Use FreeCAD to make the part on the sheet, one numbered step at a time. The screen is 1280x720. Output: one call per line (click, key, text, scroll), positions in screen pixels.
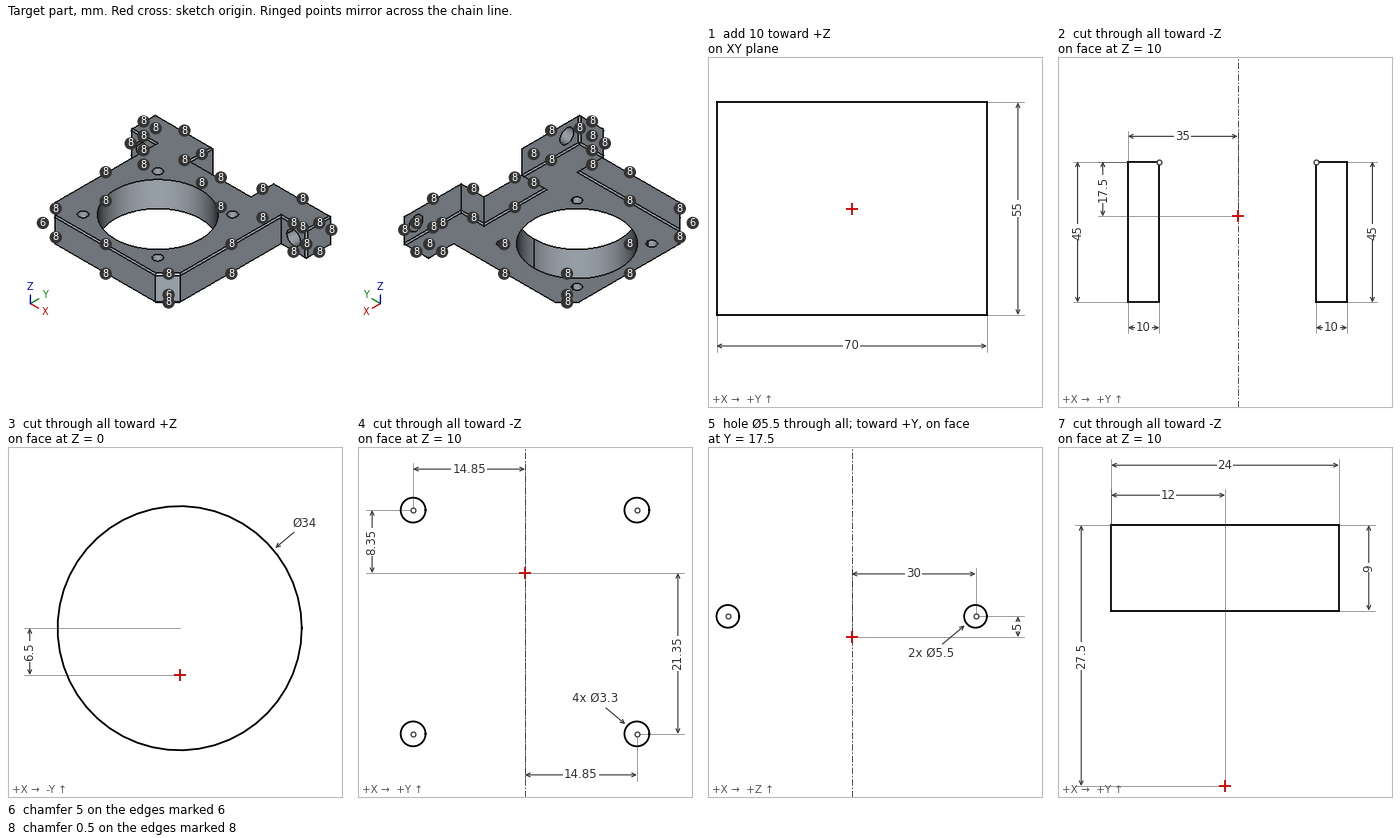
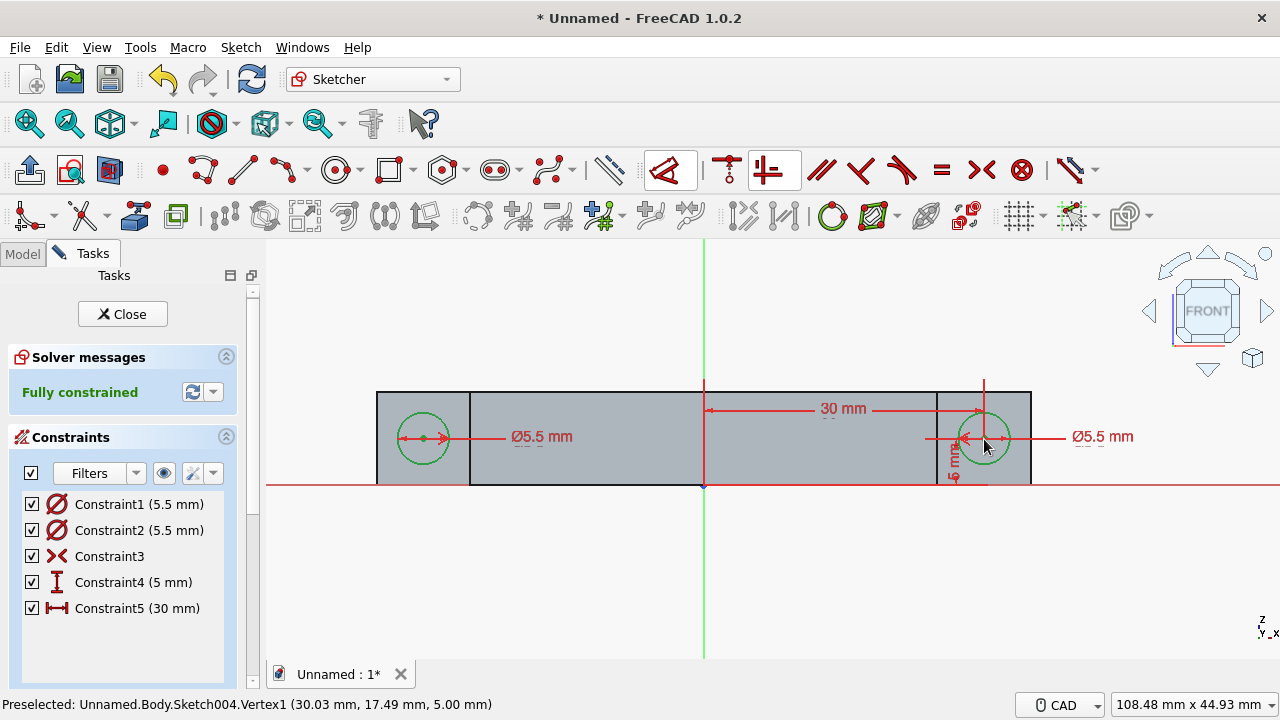
click(123, 314)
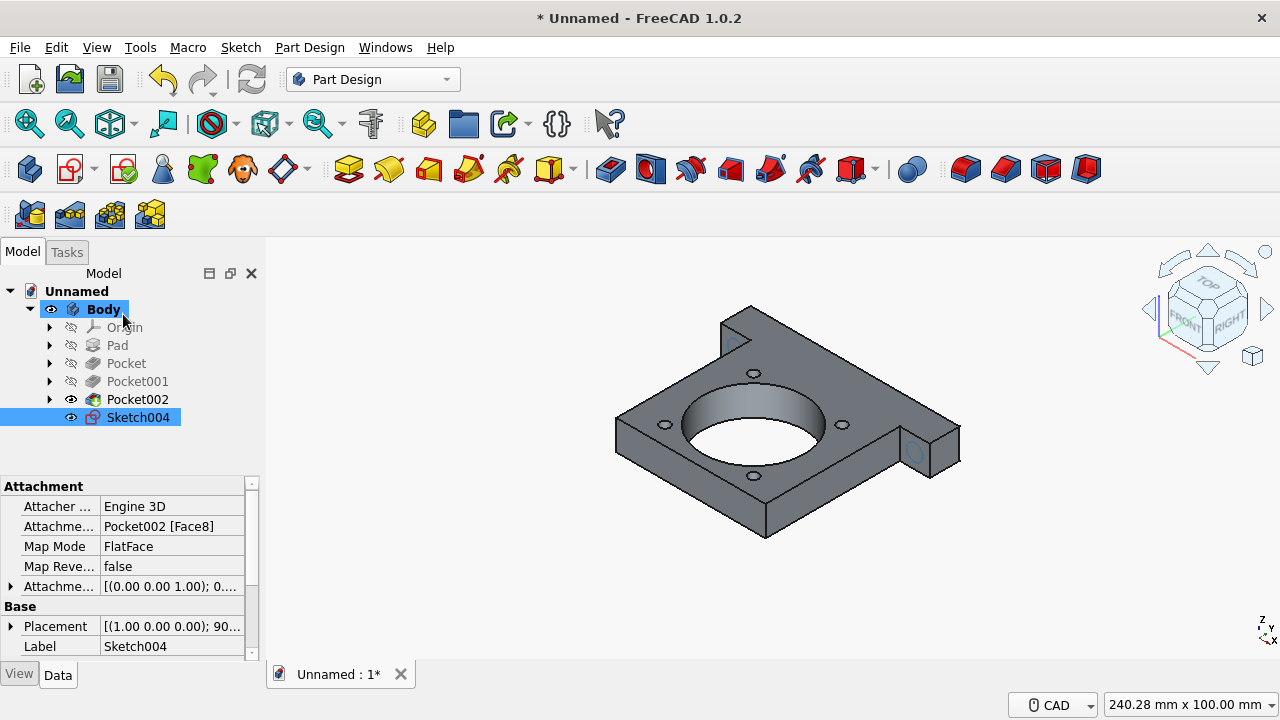
click(652, 170)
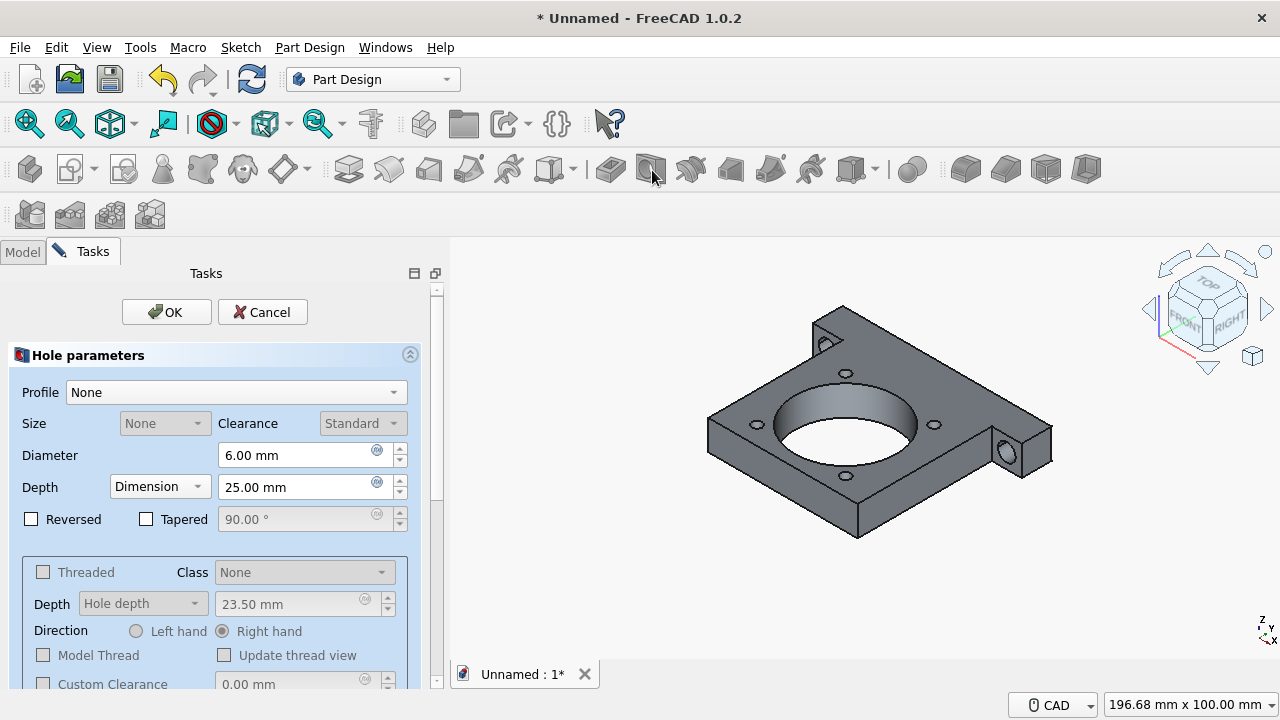
triple_click(305, 455)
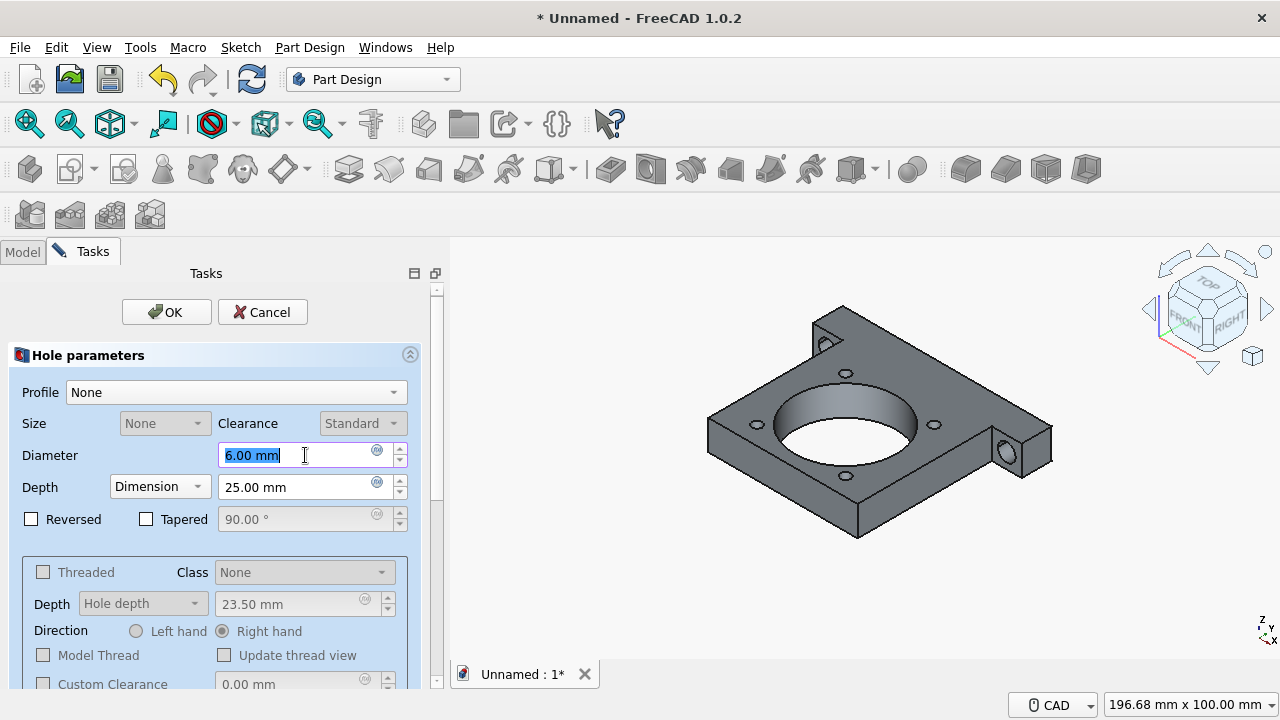
text(5.5)
key(Tab)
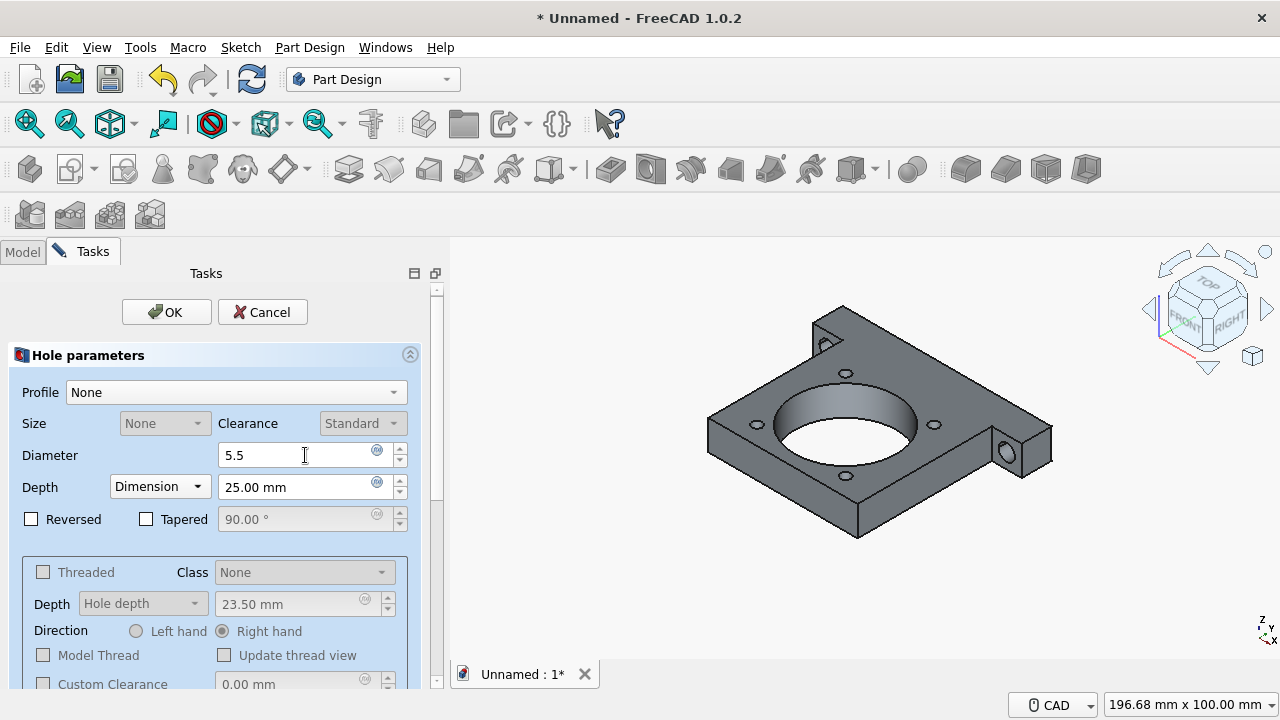
click(161, 486)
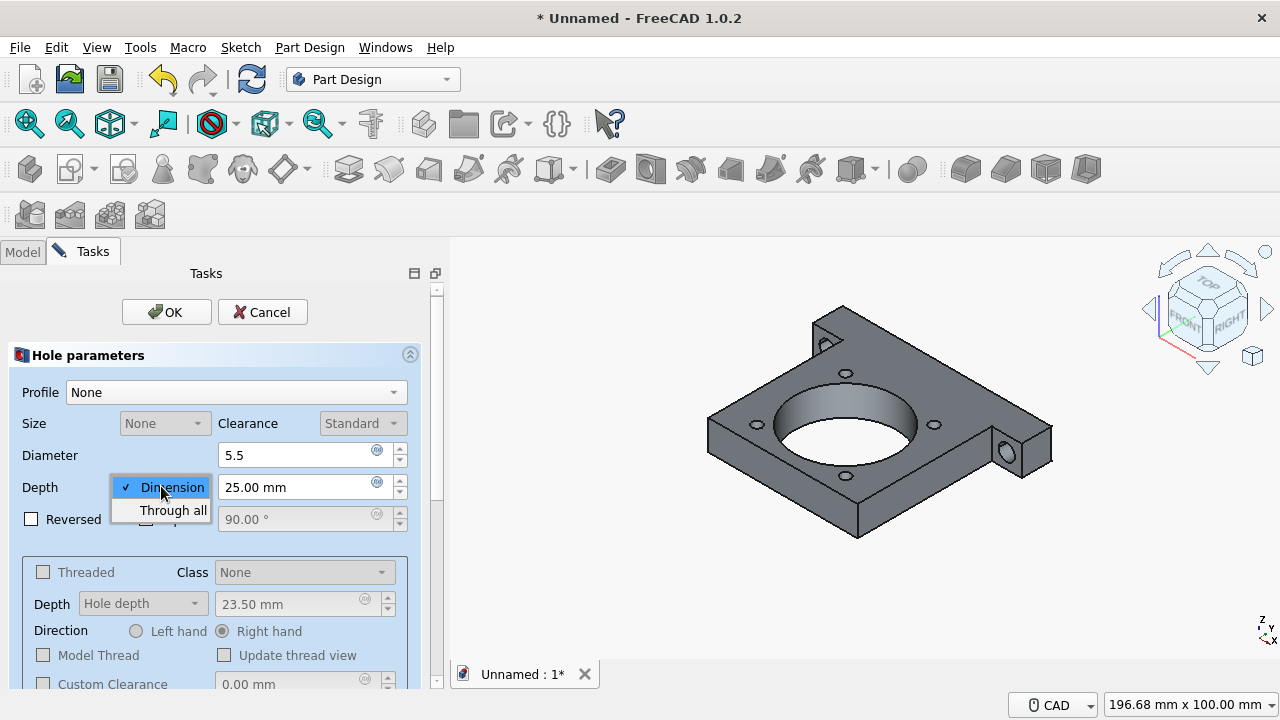
click(160, 510)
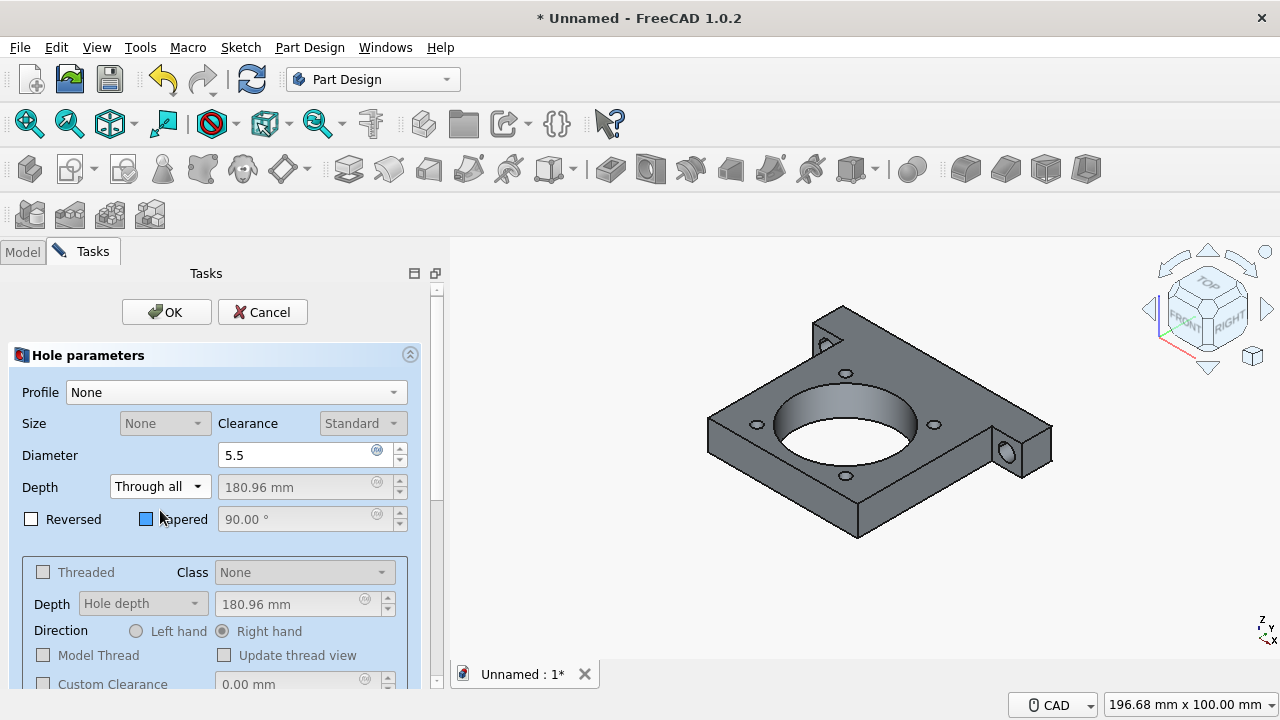
click(167, 312)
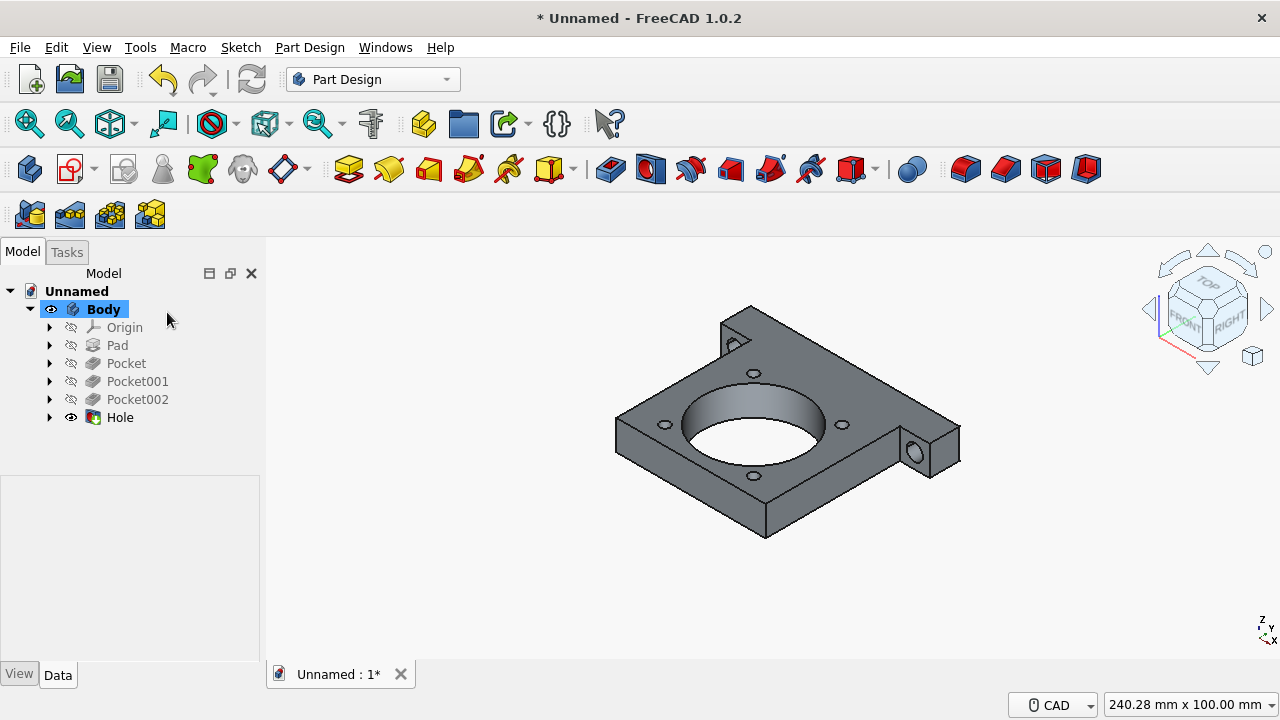
click(766, 520)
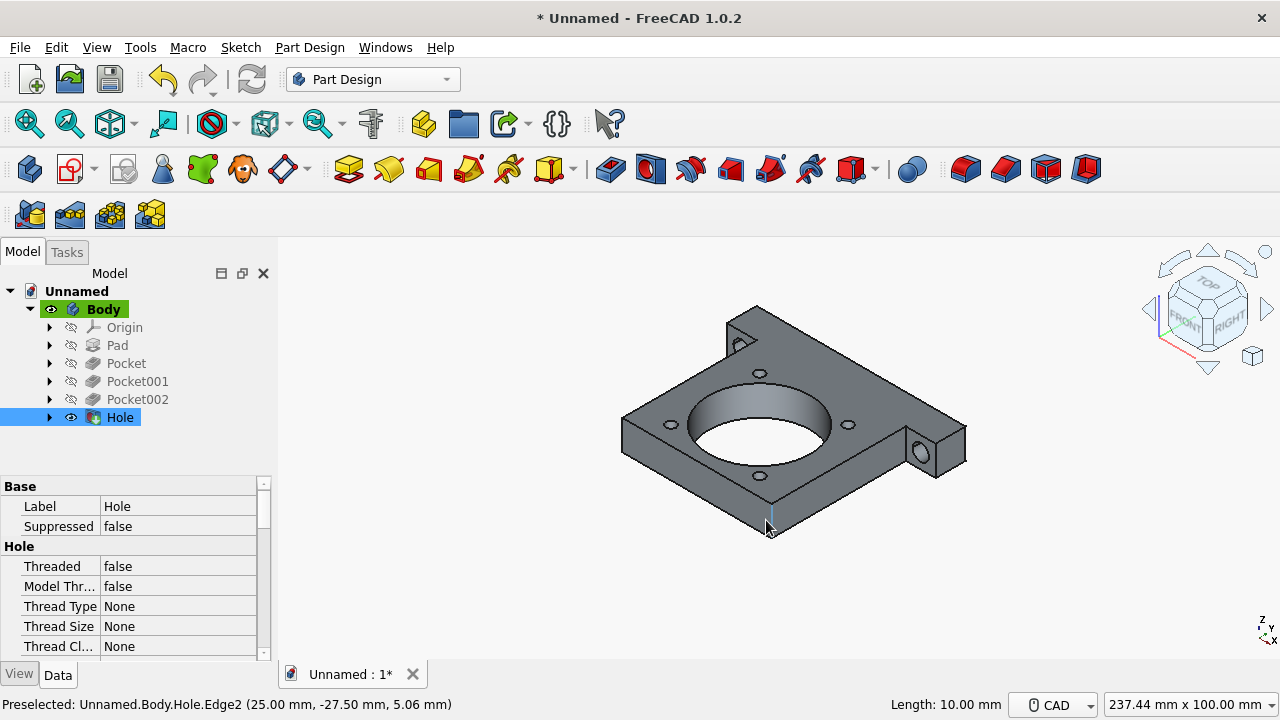
key(2)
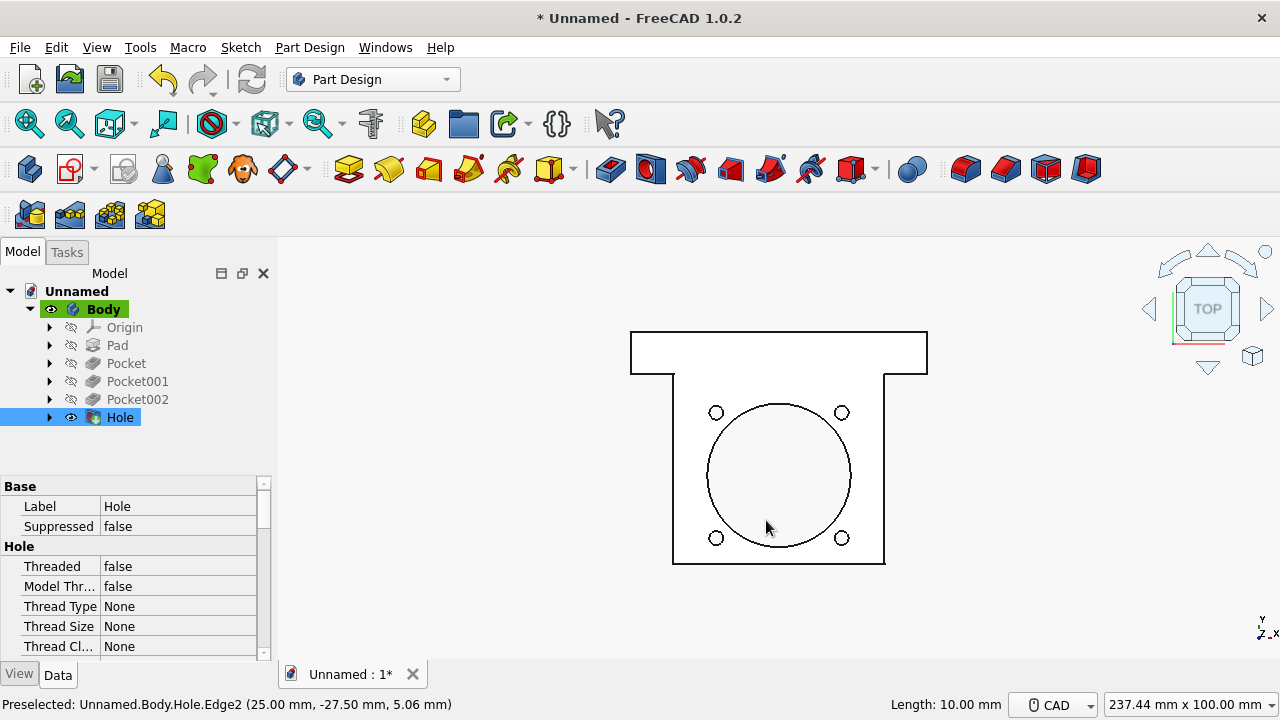
key(0)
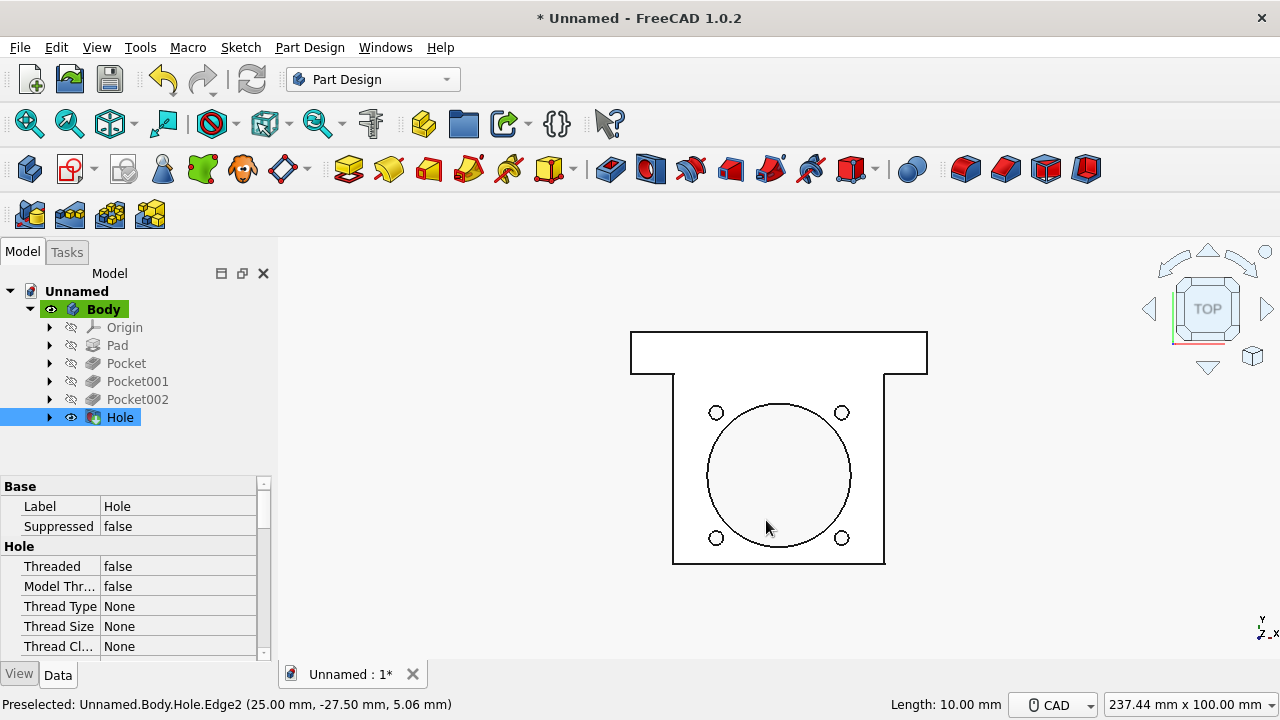
key(1)